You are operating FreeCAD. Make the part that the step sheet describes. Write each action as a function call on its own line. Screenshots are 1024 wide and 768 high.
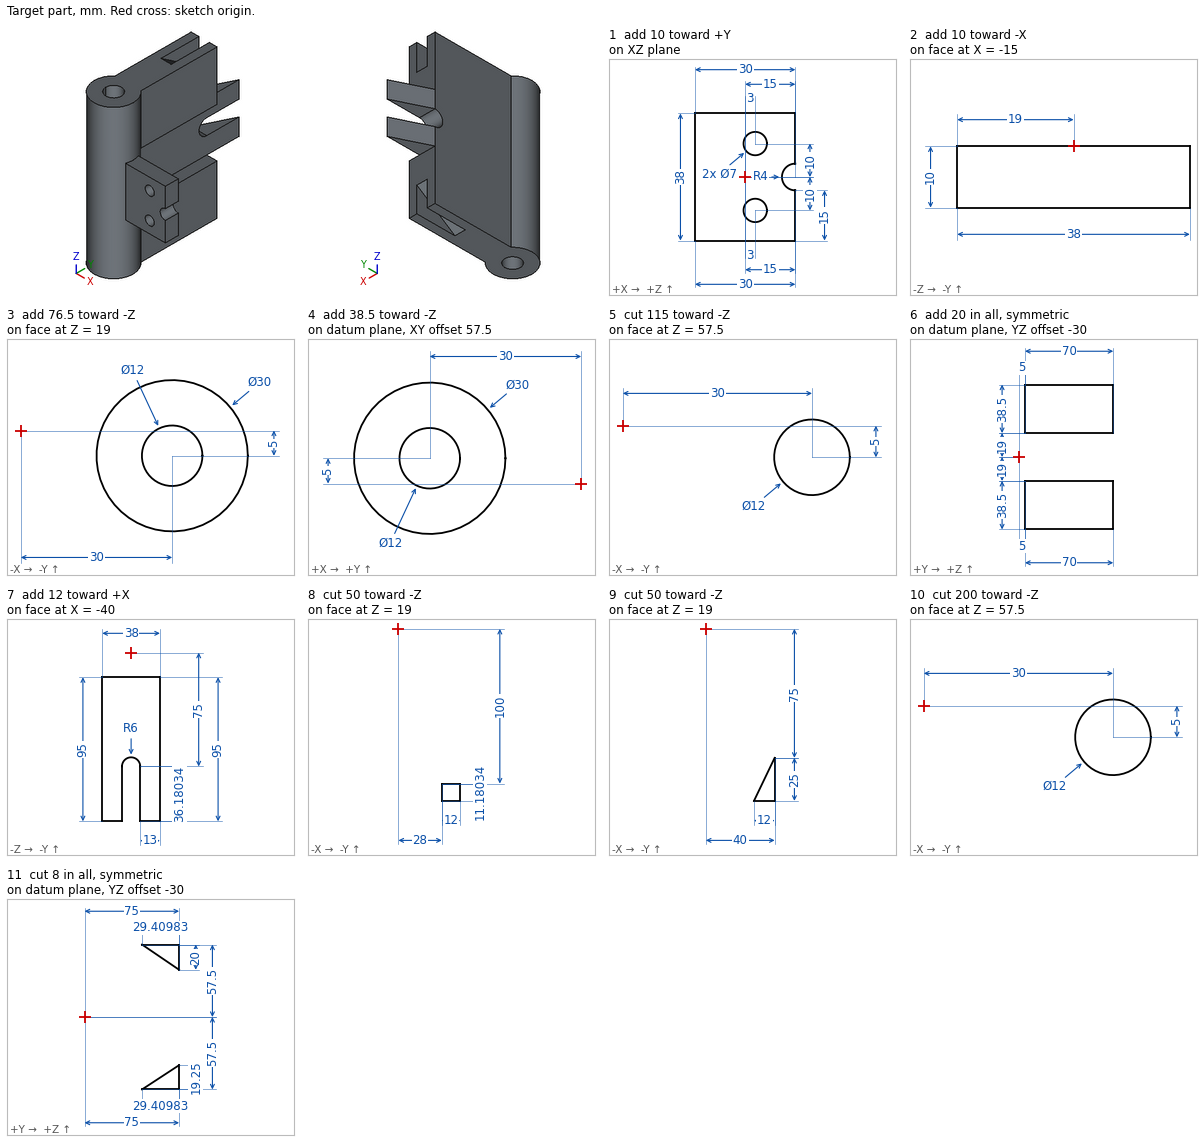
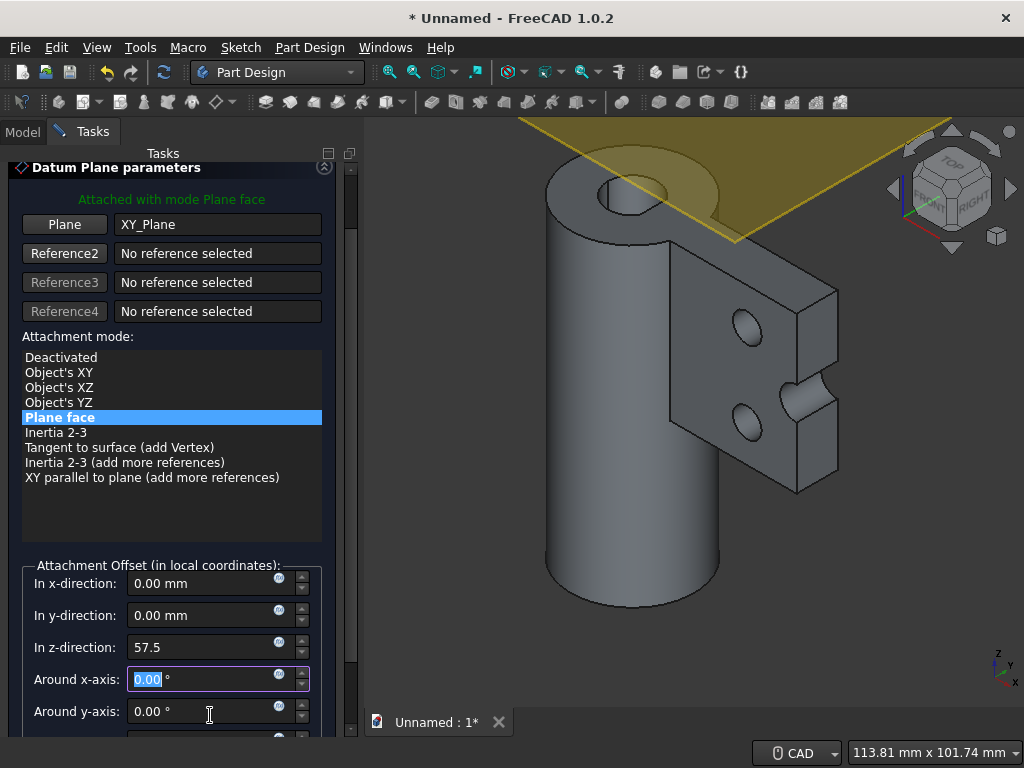
scroll(351, 450, up, 2)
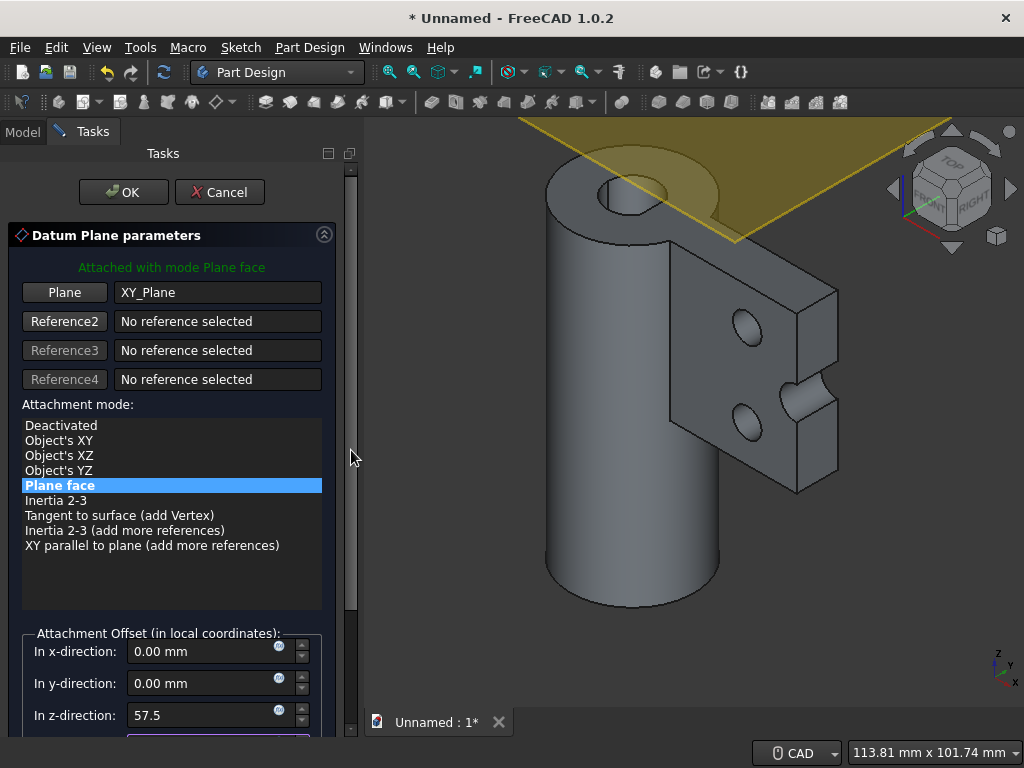
click(124, 192)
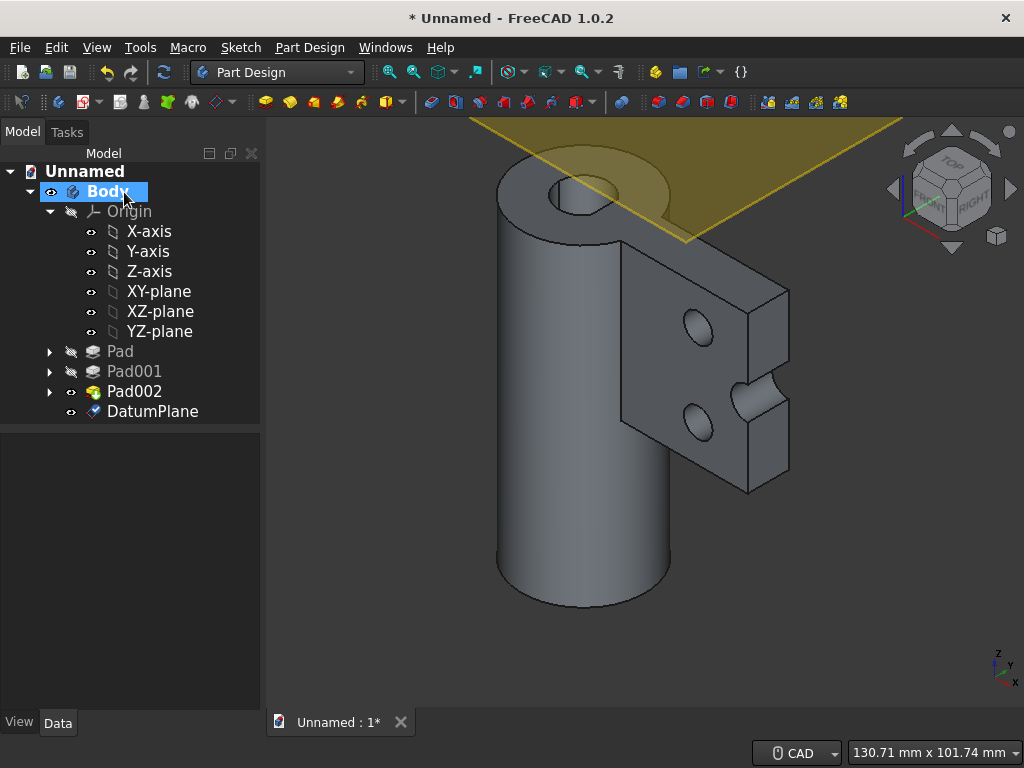
click(116, 412)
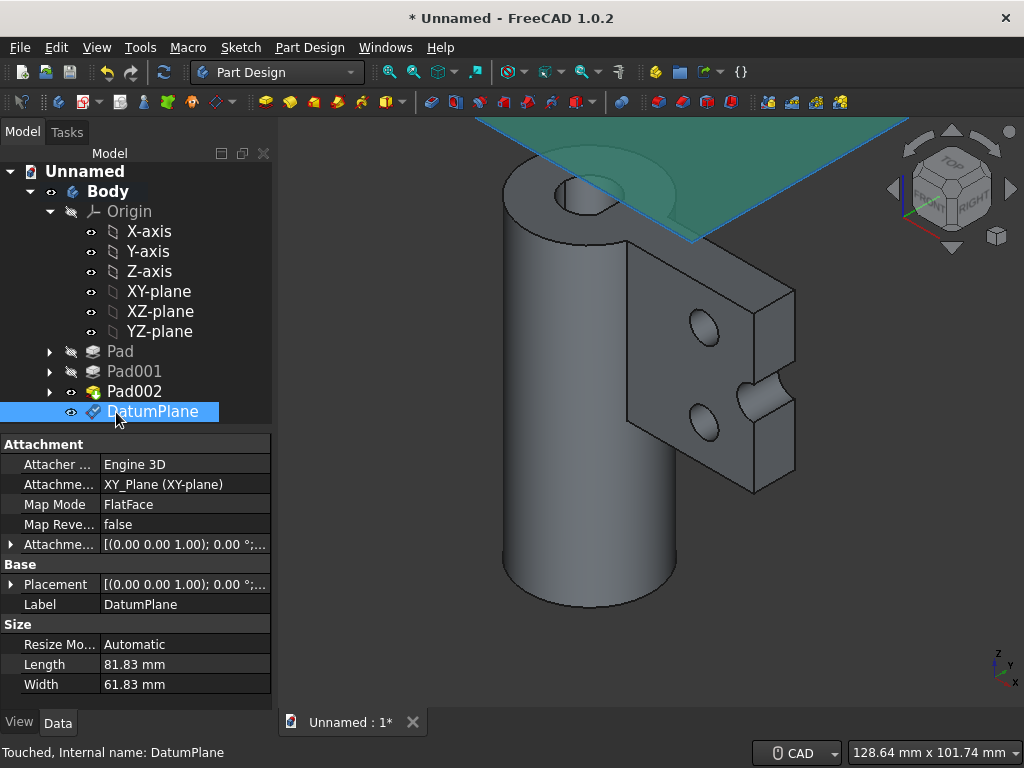
click(84, 102)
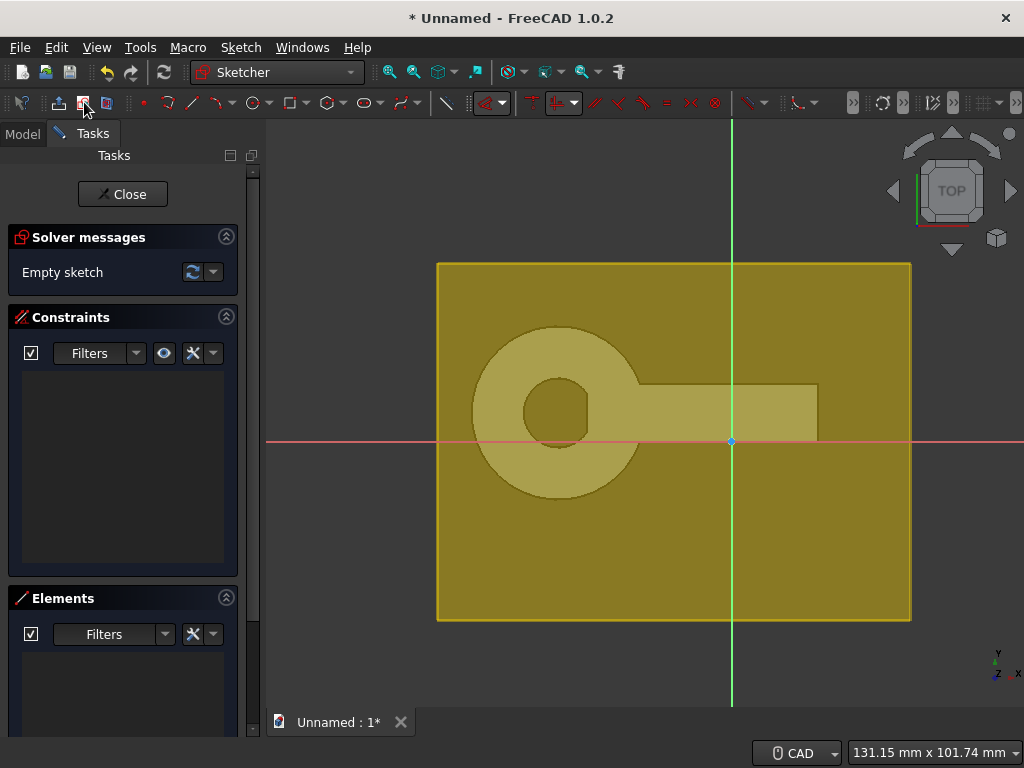
scroll(653, 413, up, 2)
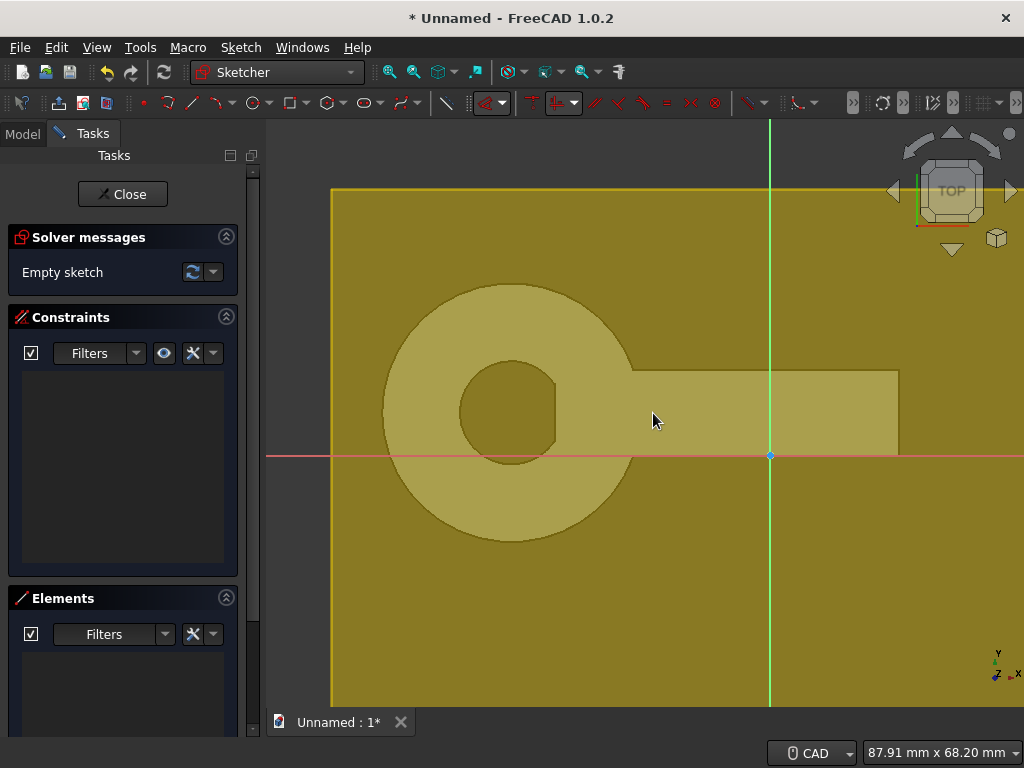
click(254, 104)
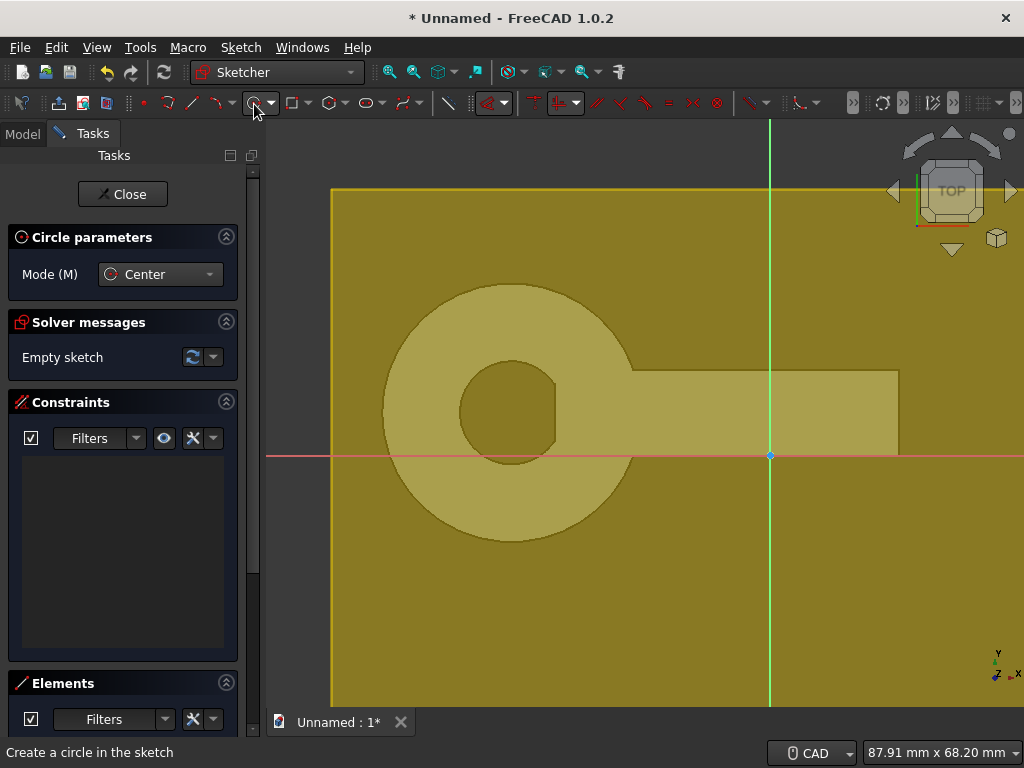
click(511, 413)
click(603, 321)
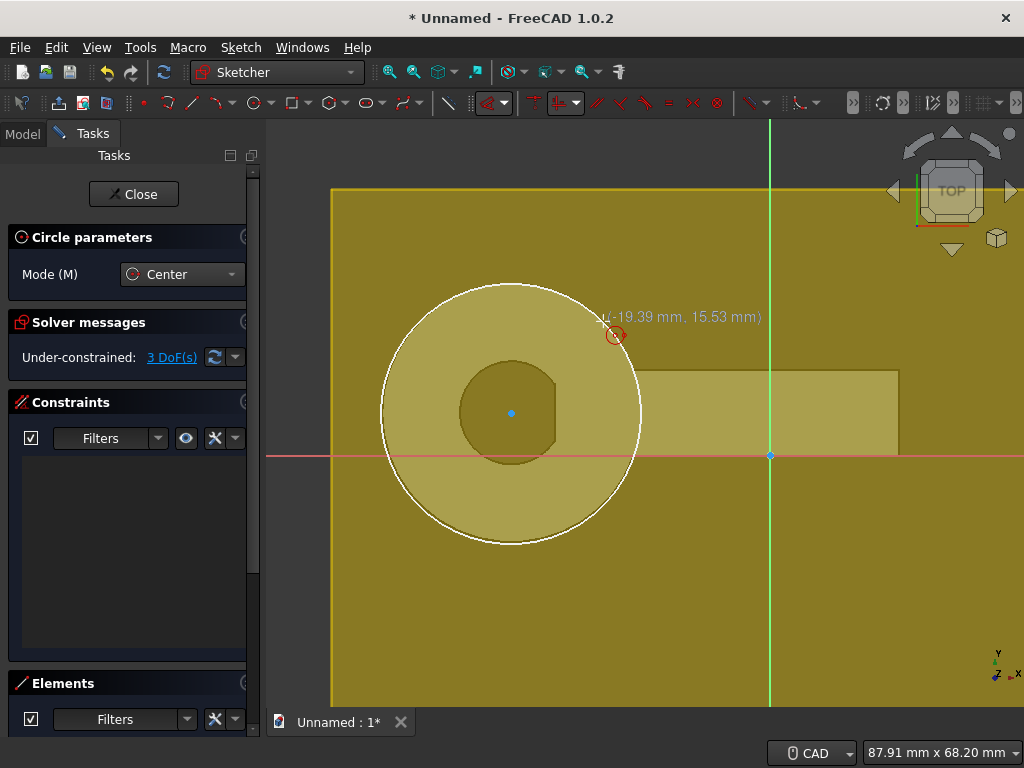
click(511, 414)
click(548, 376)
key(Escape)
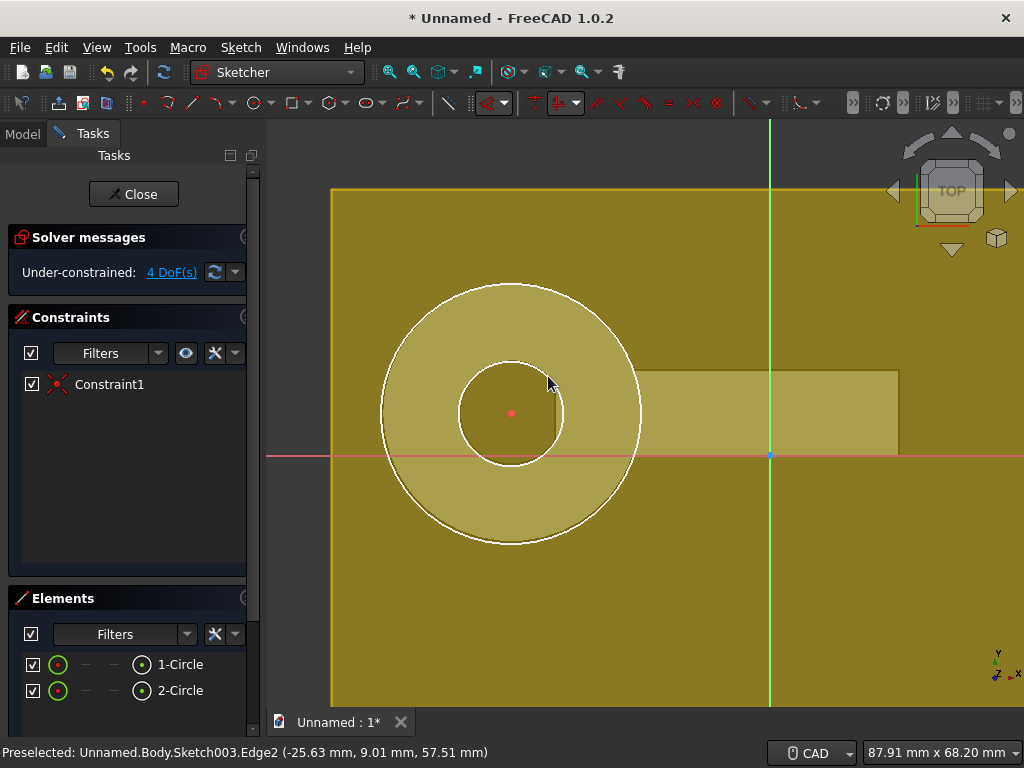
click(603, 322)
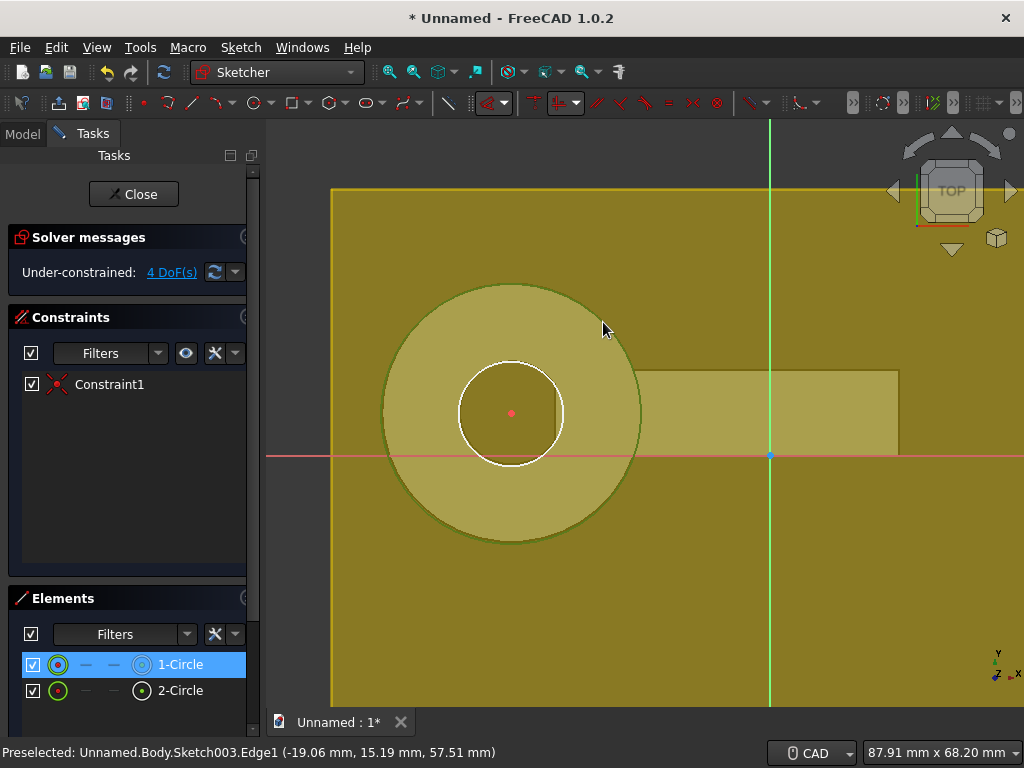
click(506, 104)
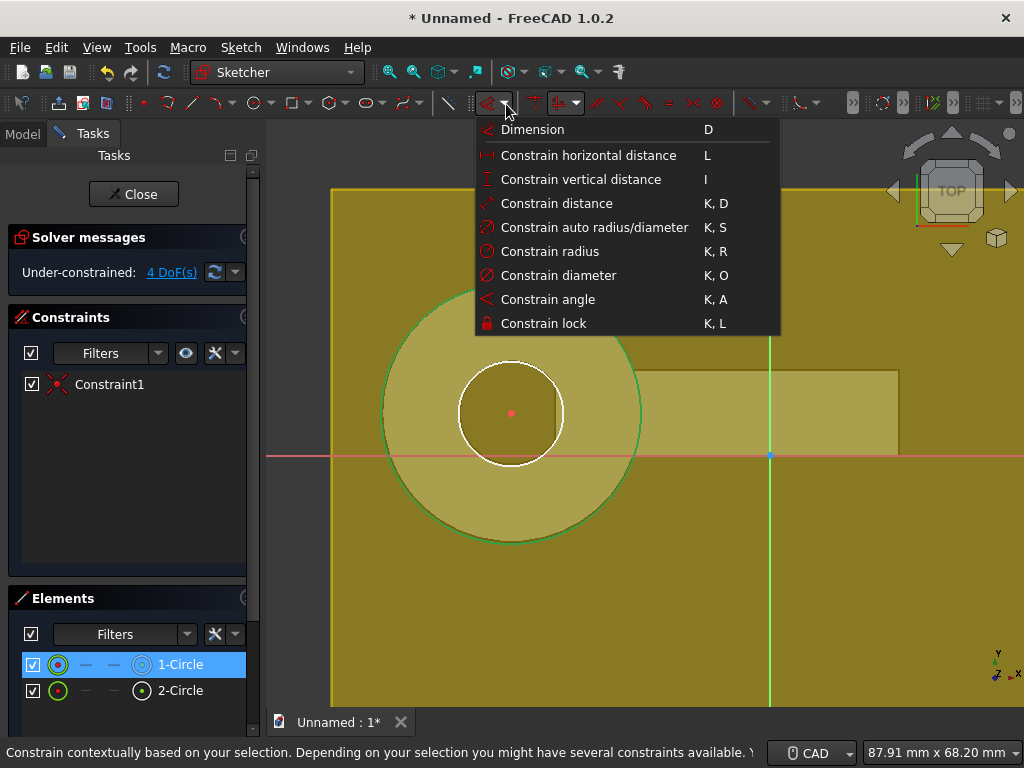
click(628, 275)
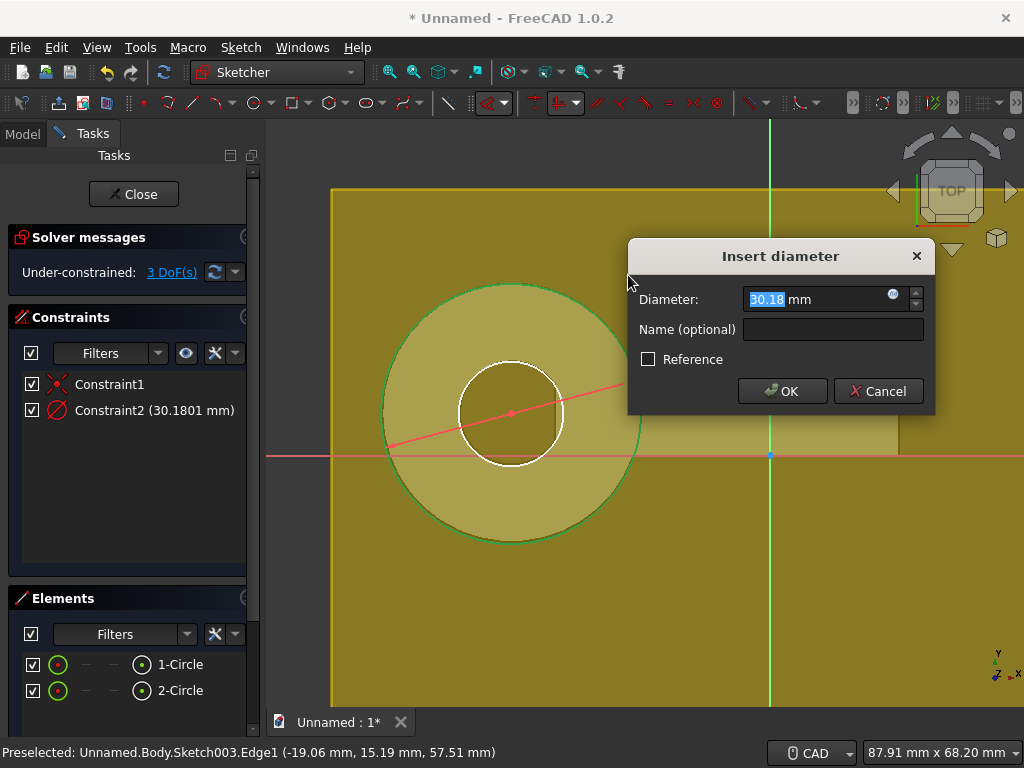
text(30)
key(Return)